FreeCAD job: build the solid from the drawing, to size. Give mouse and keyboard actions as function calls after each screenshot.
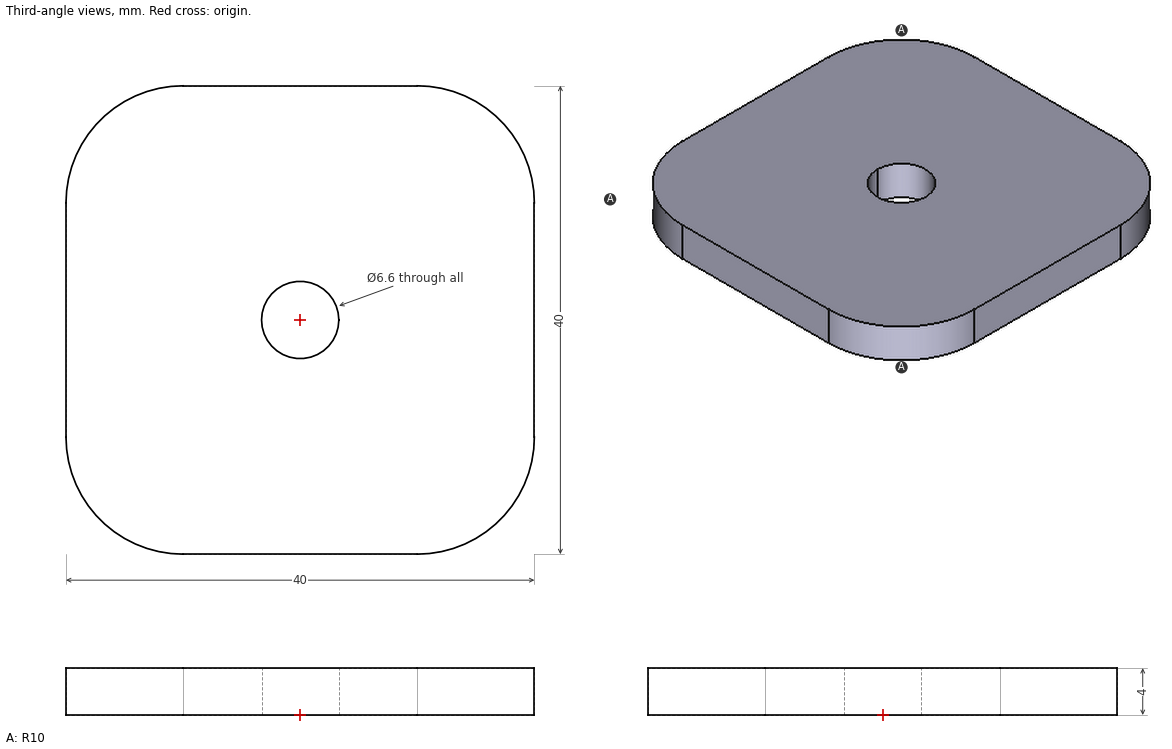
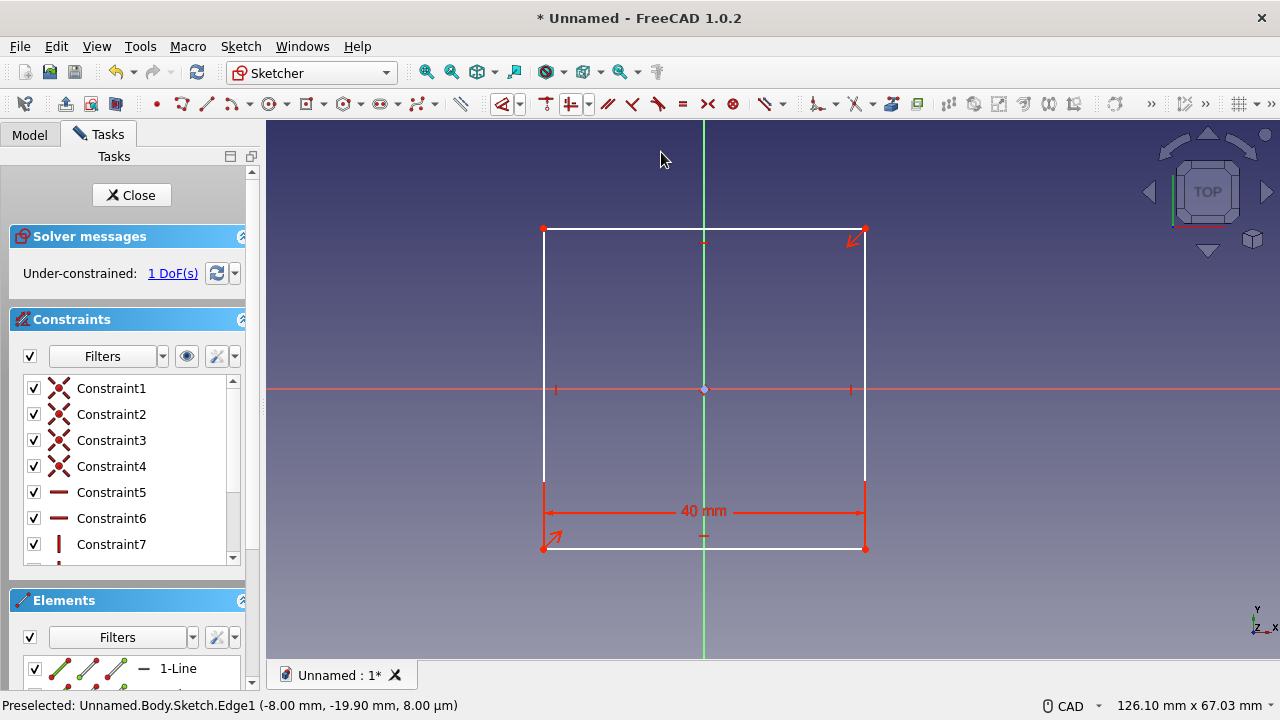
click(865, 453)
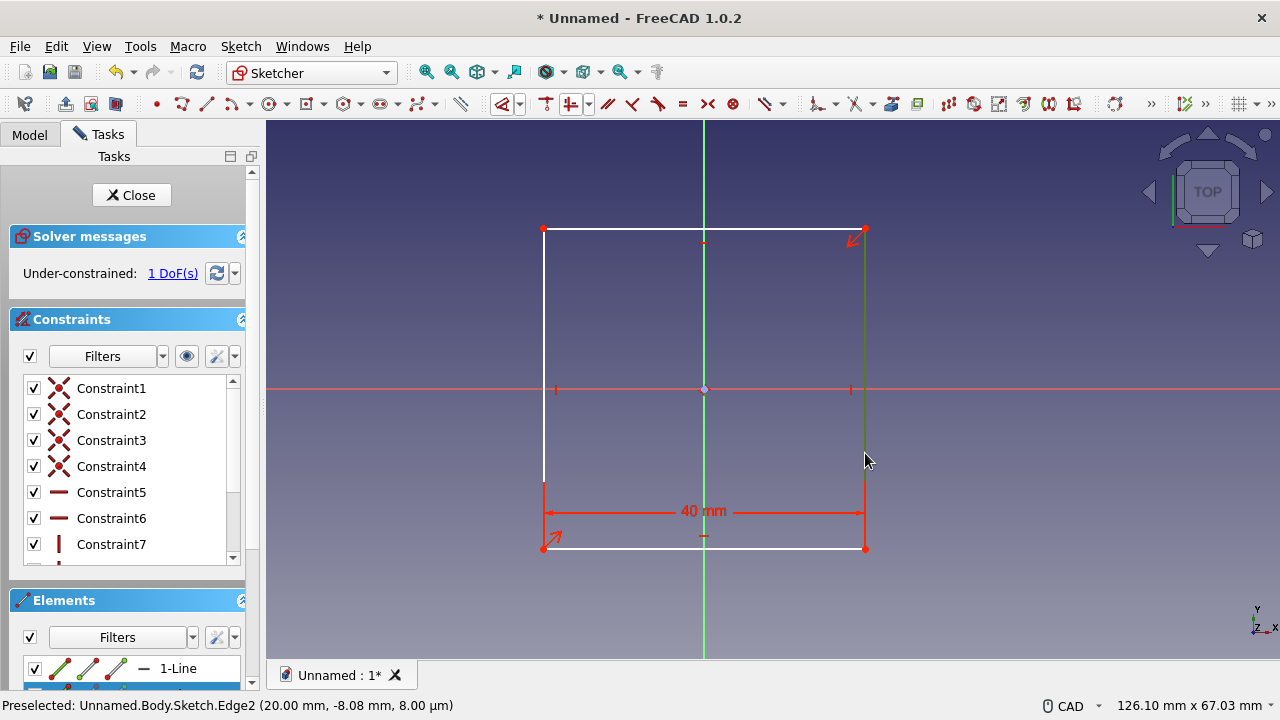
key(i)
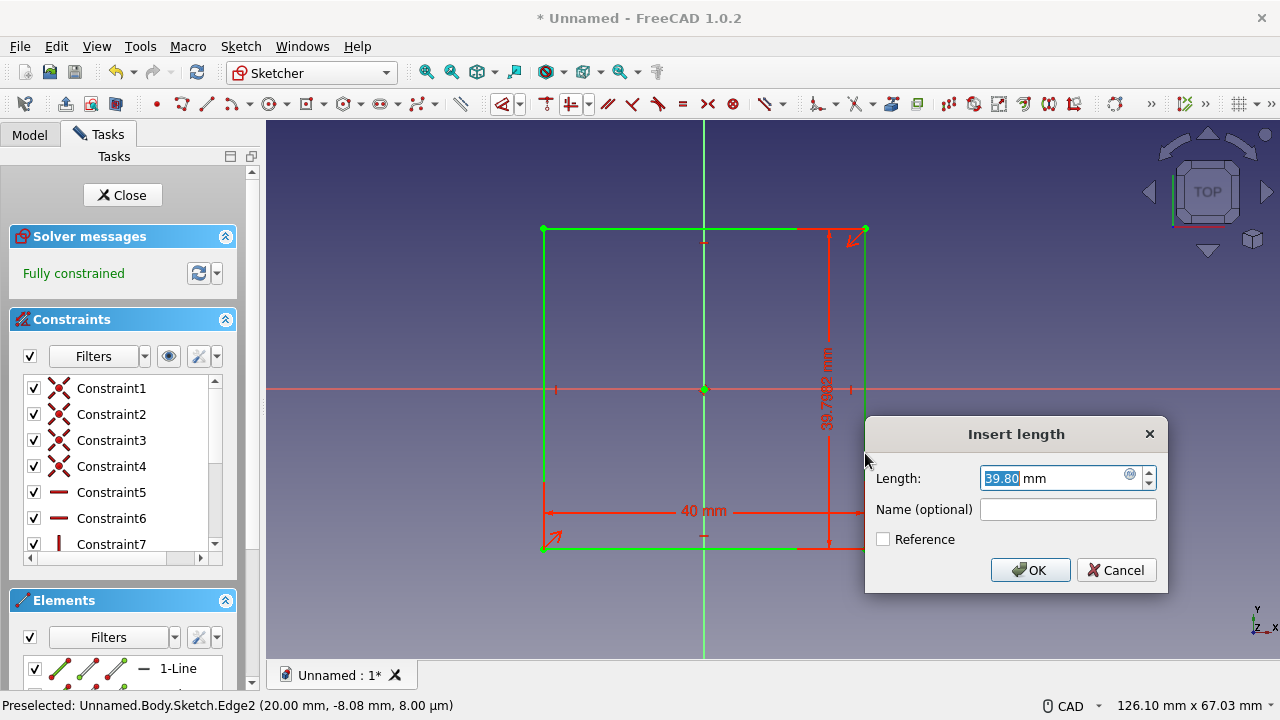
text(40)
key(Return)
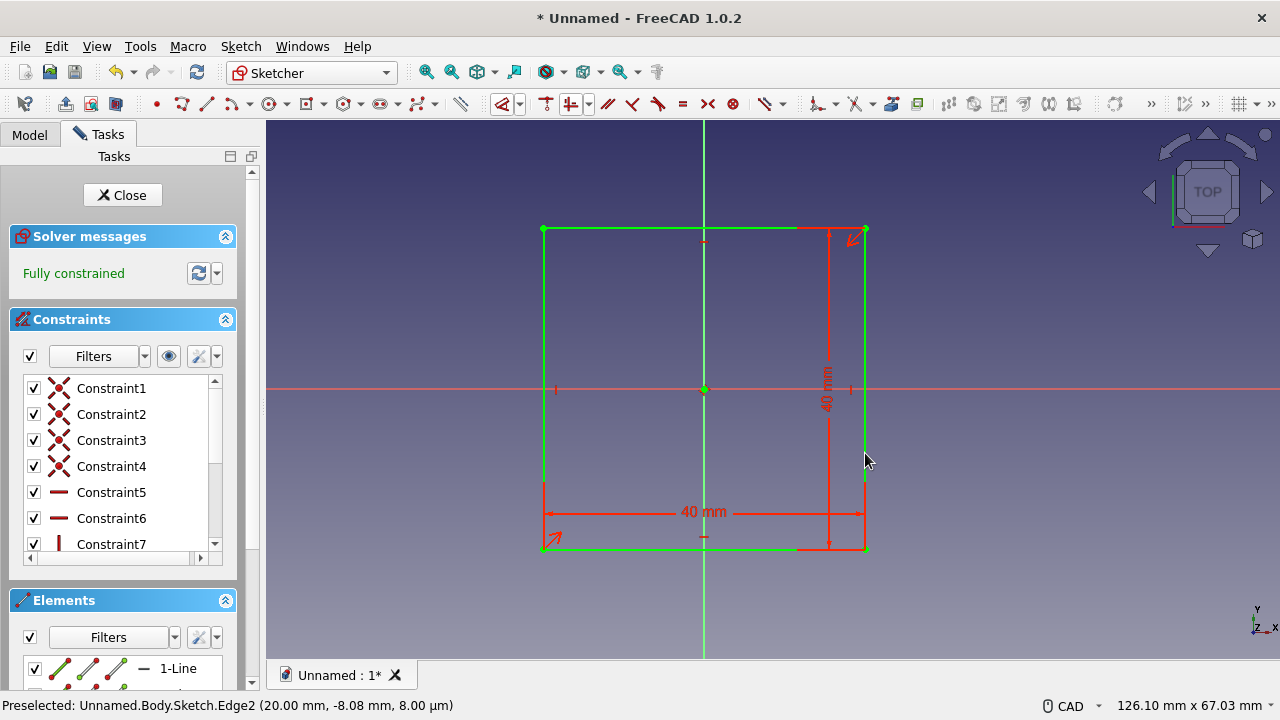
click(123, 195)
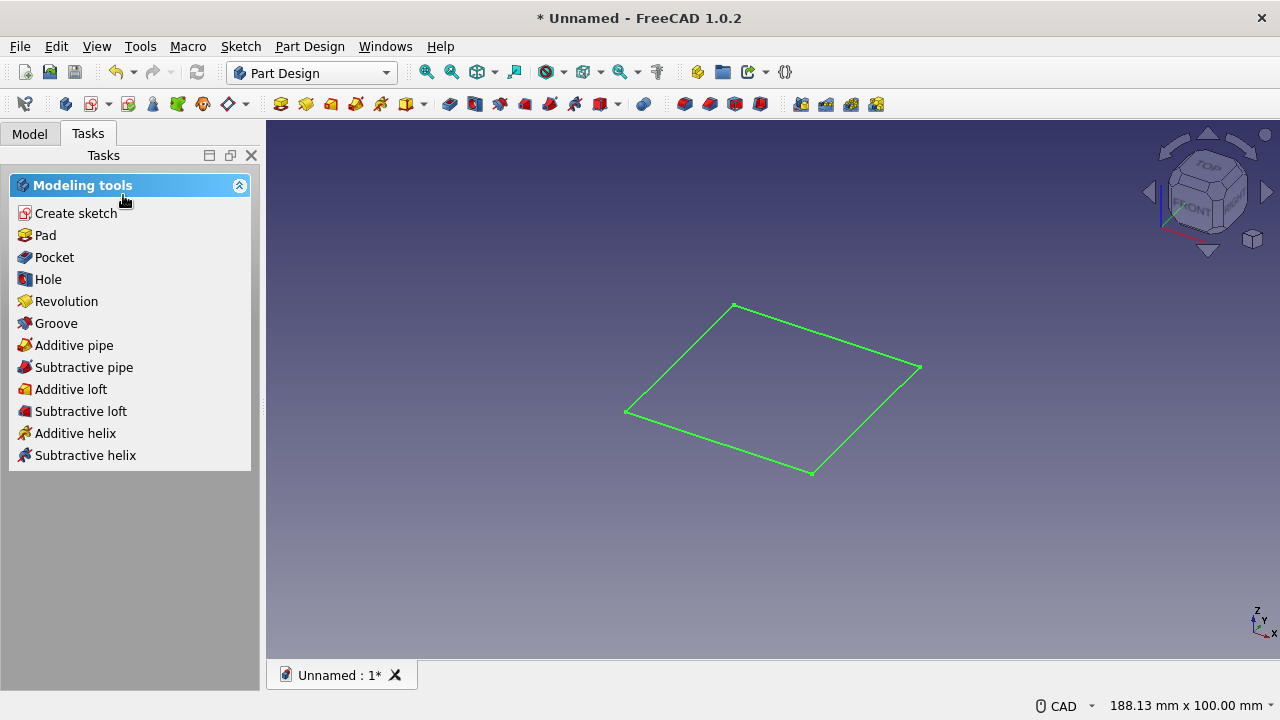
click(281, 104)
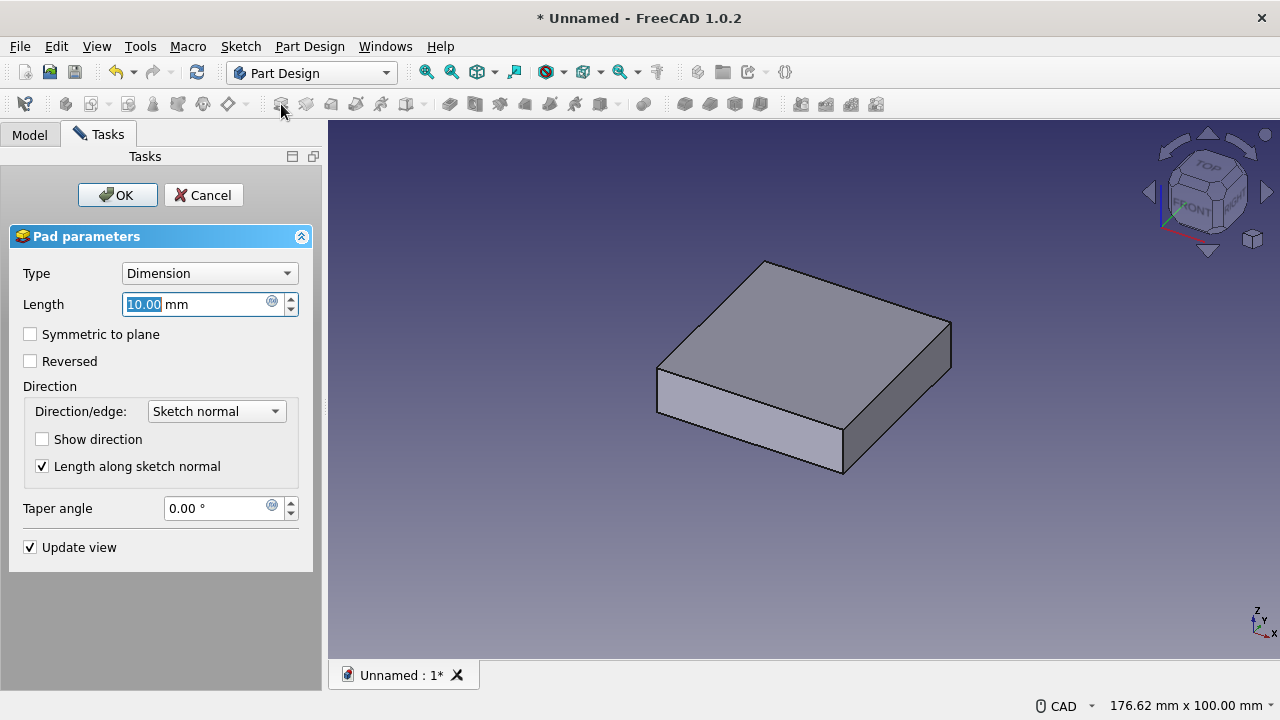
text(4)
key(Tab)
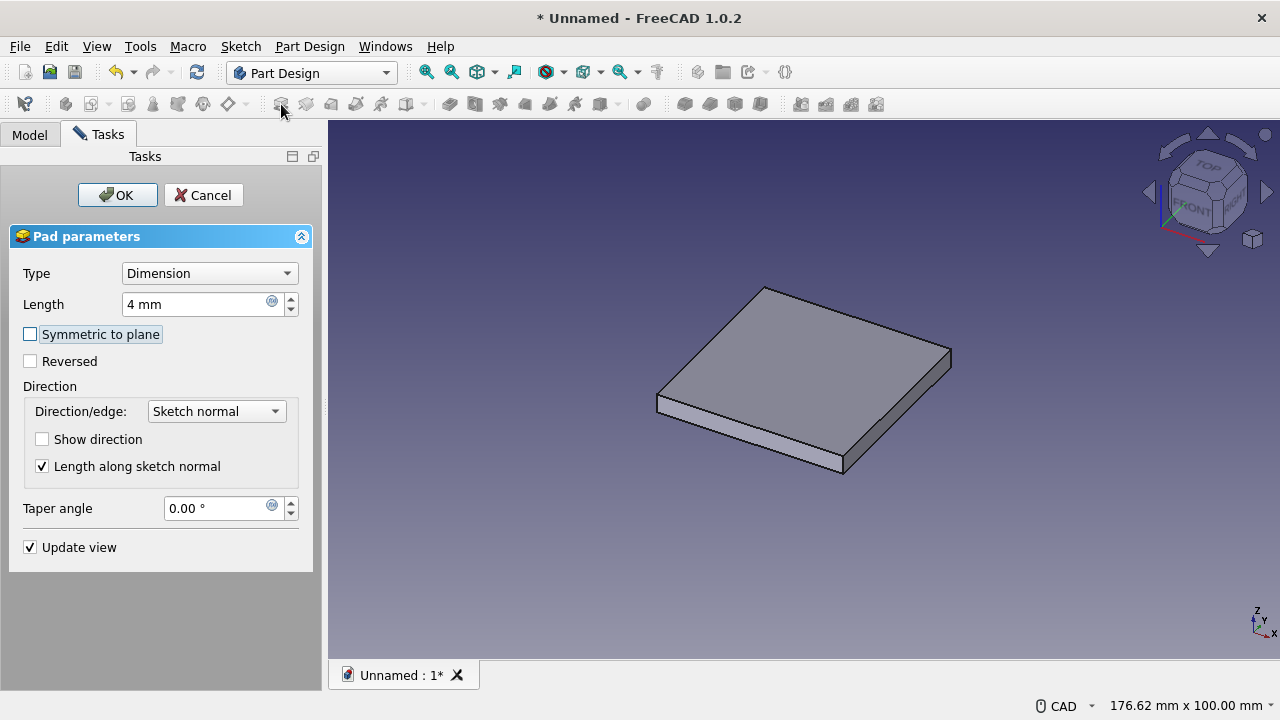
click(118, 195)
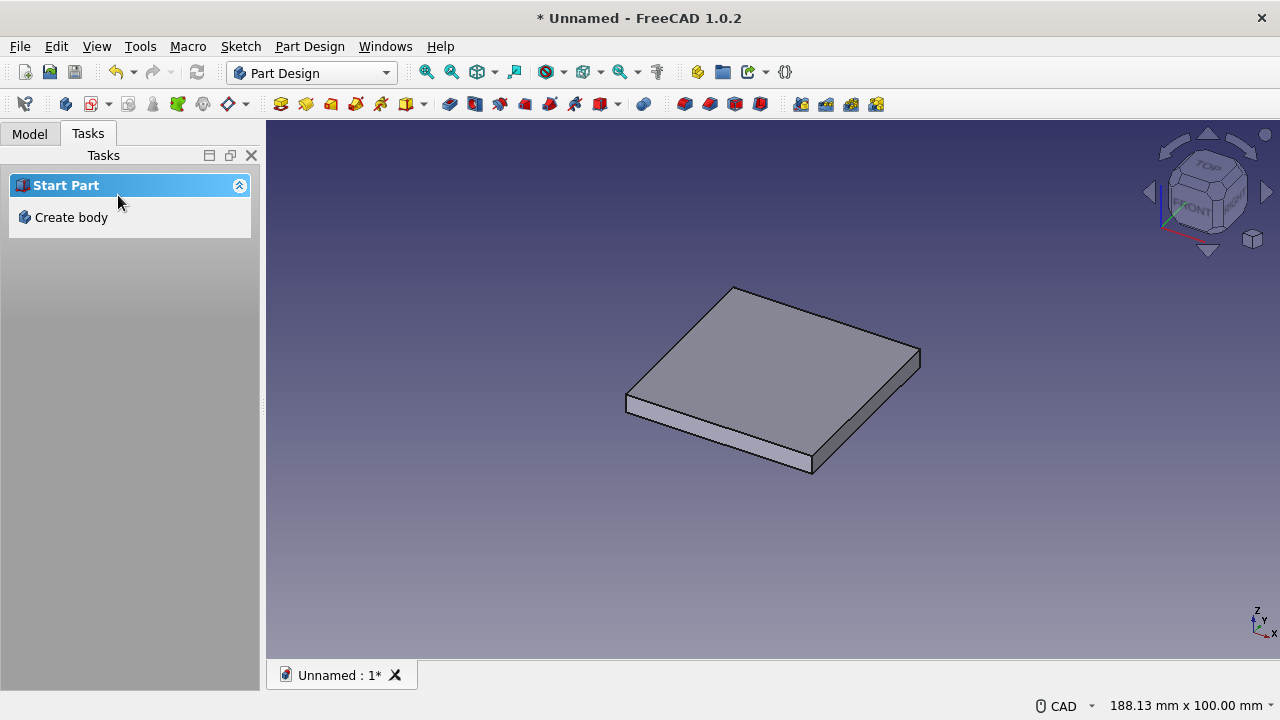
click(427, 72)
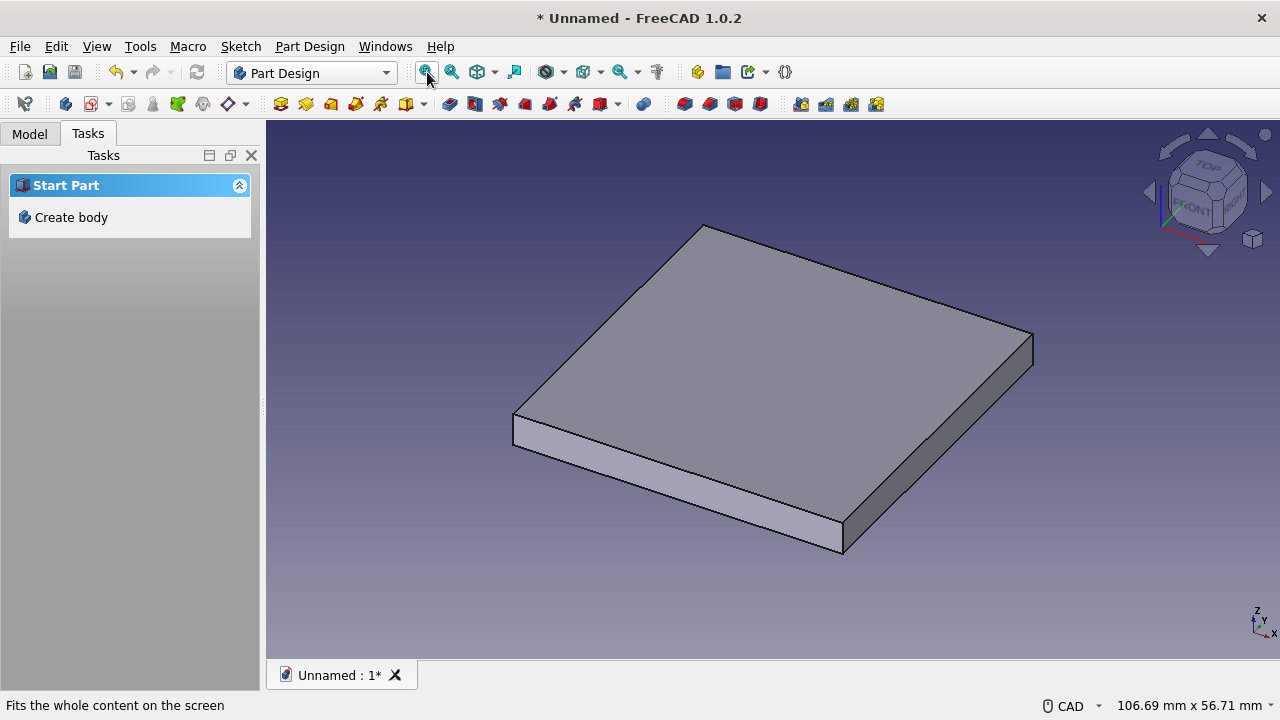
click(843, 537)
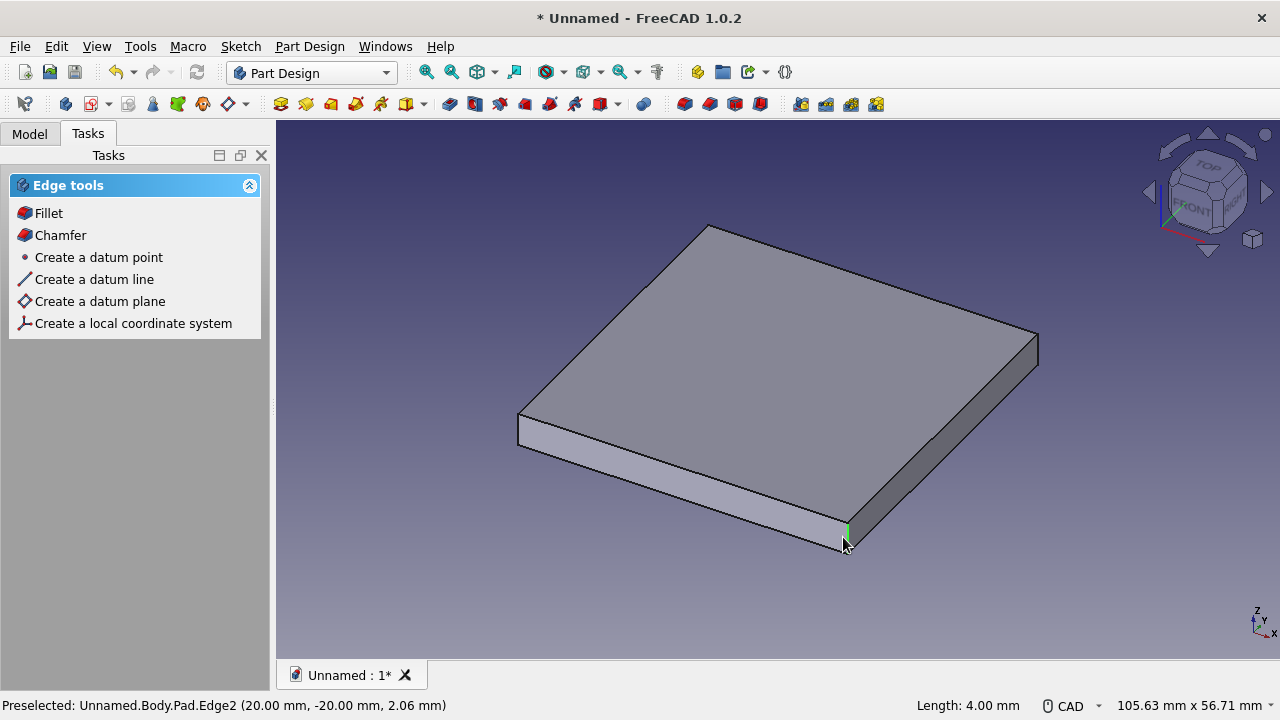
key(0)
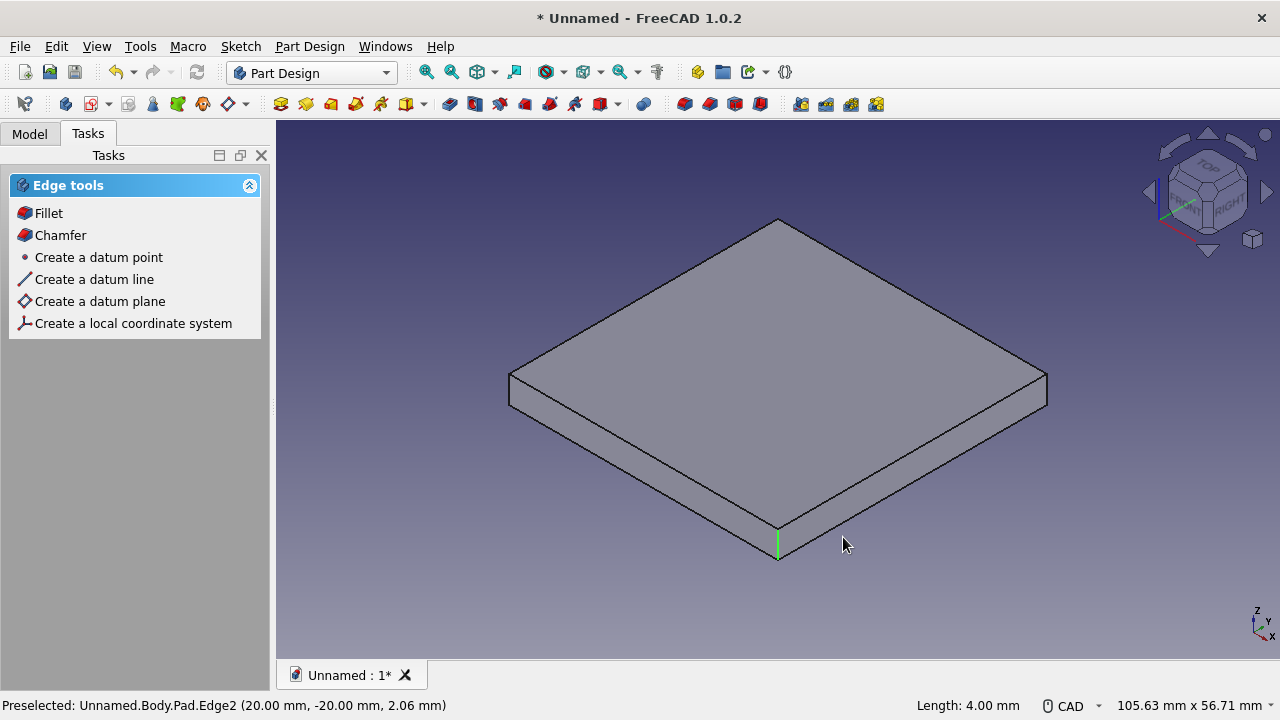
key(2)